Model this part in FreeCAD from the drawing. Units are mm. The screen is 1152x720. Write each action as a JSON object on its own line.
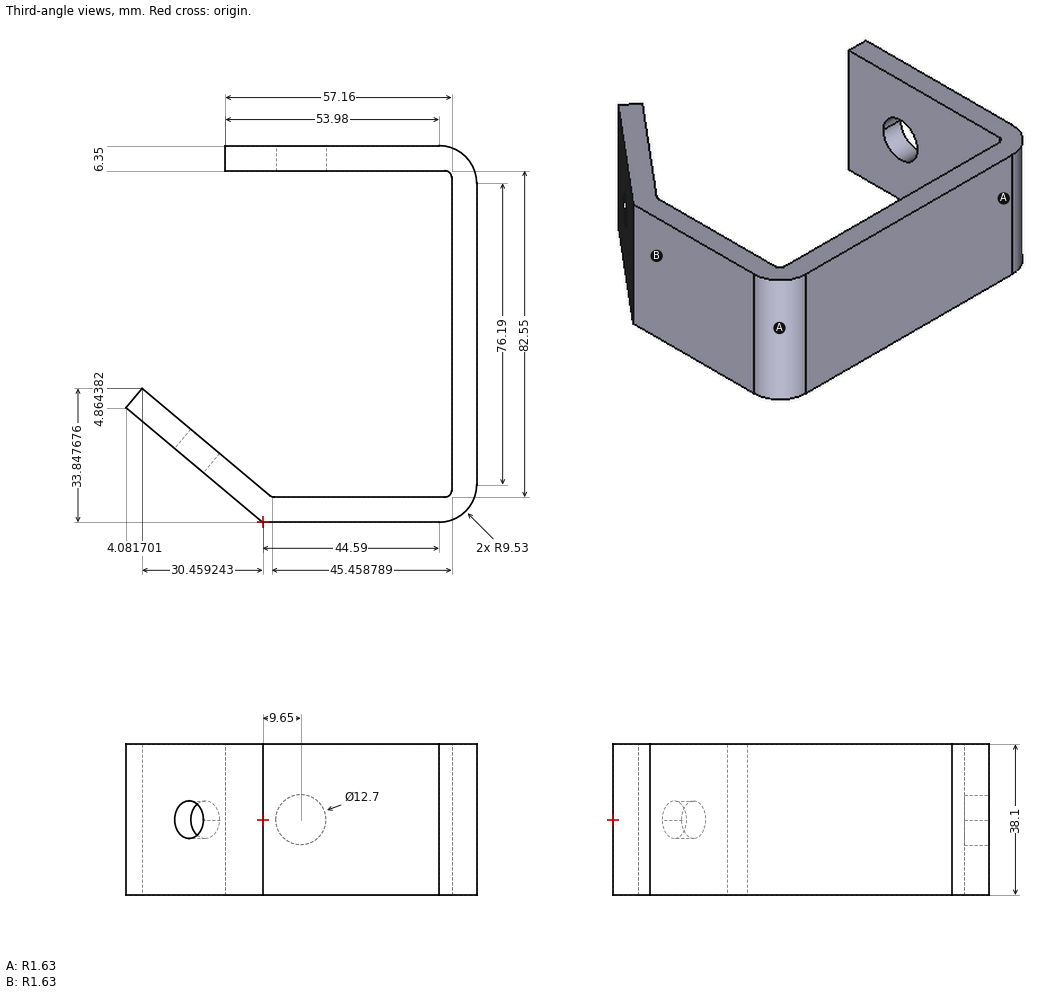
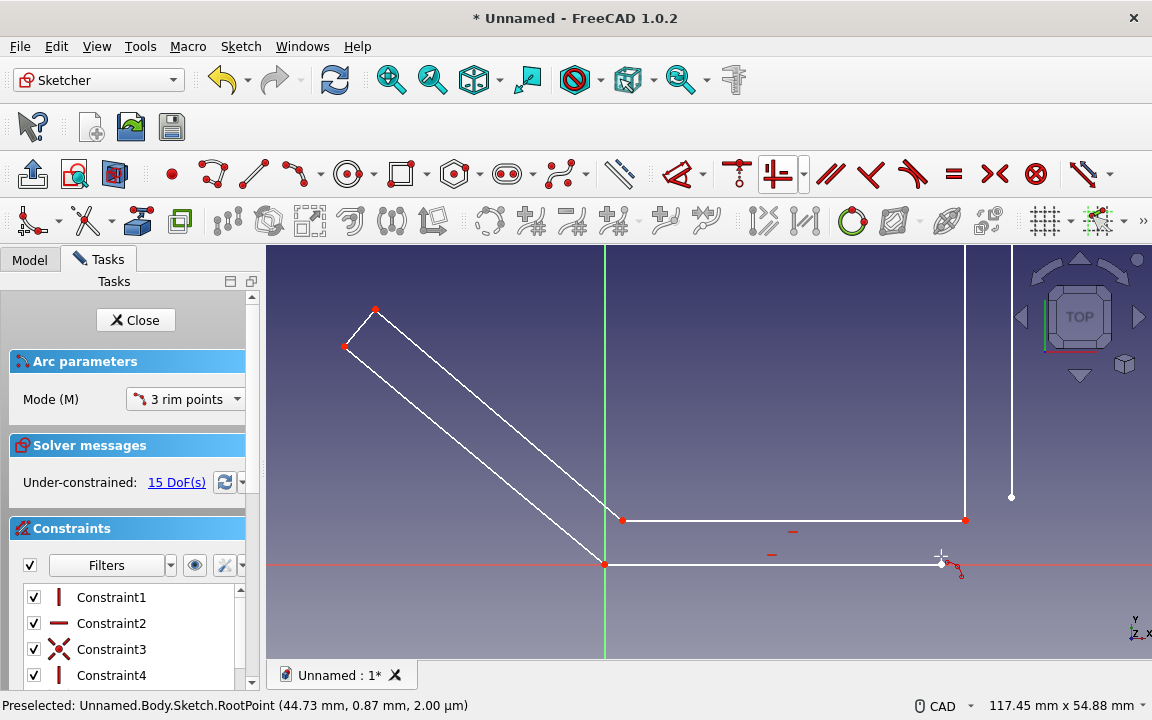
{"action": "scroll", "coordinate": [618, 596], "scroll_direction": "down", "scroll_amount": 5}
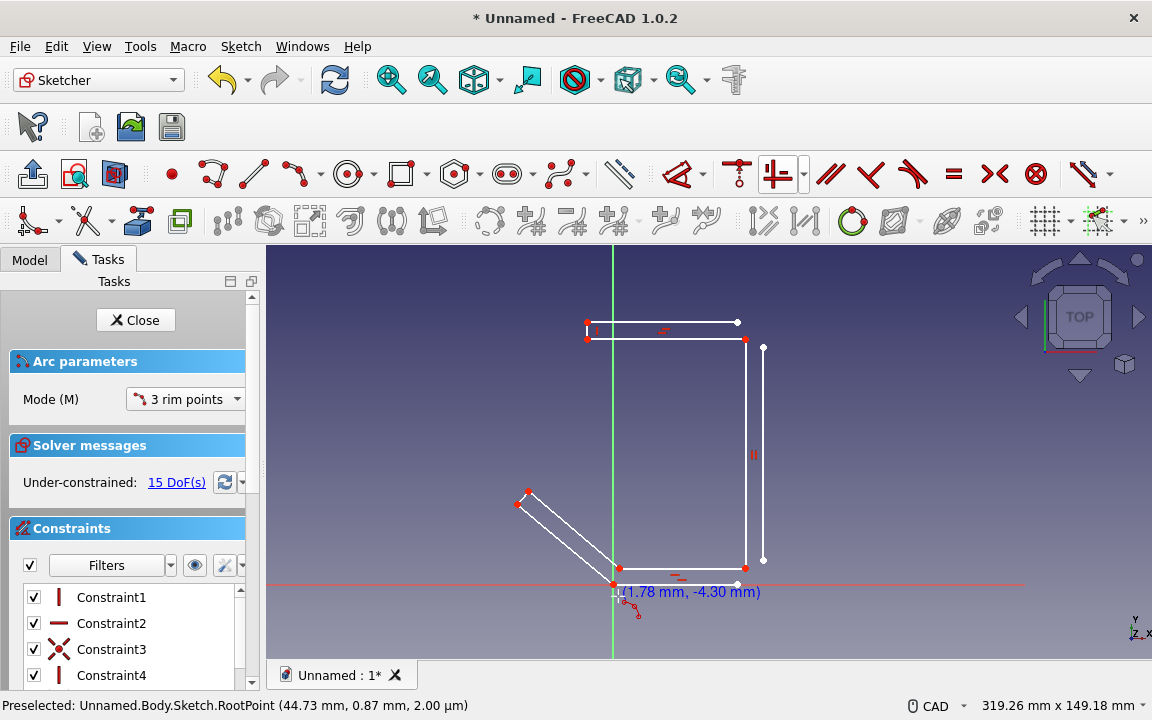
{"action": "left_click", "coordinate": [763, 348]}
{"action": "left_click", "coordinate": [737, 322]}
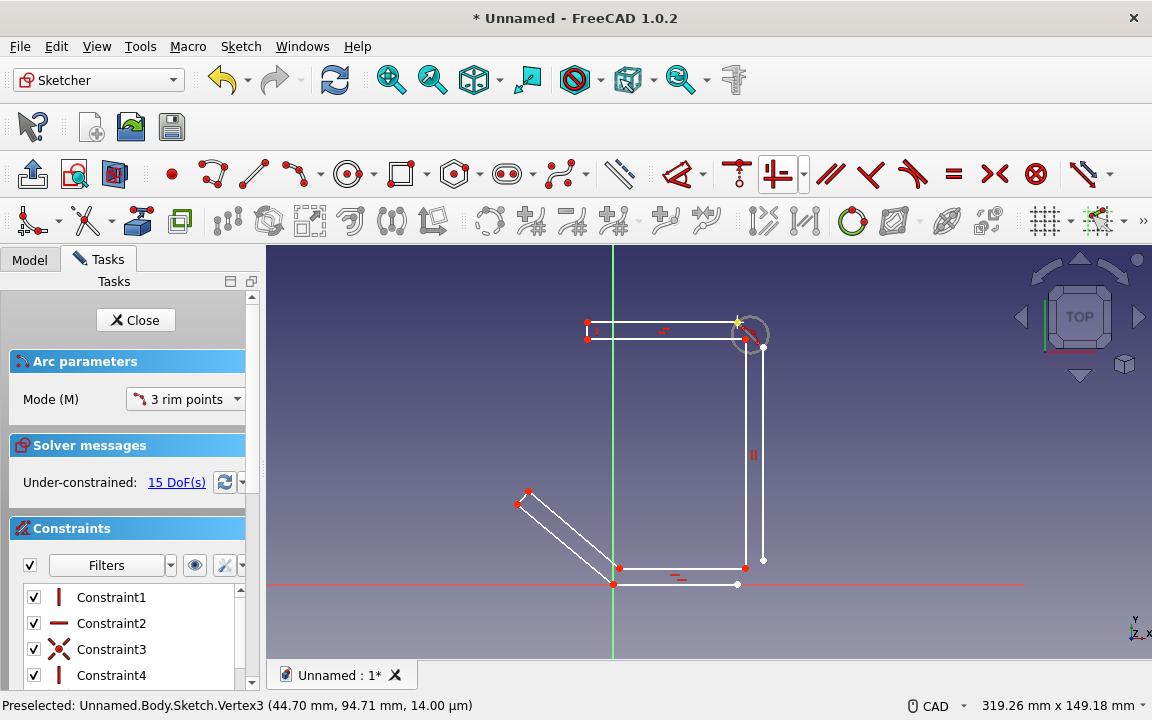
{"action": "scroll", "coordinate": [756, 328], "scroll_direction": "up", "scroll_amount": 4}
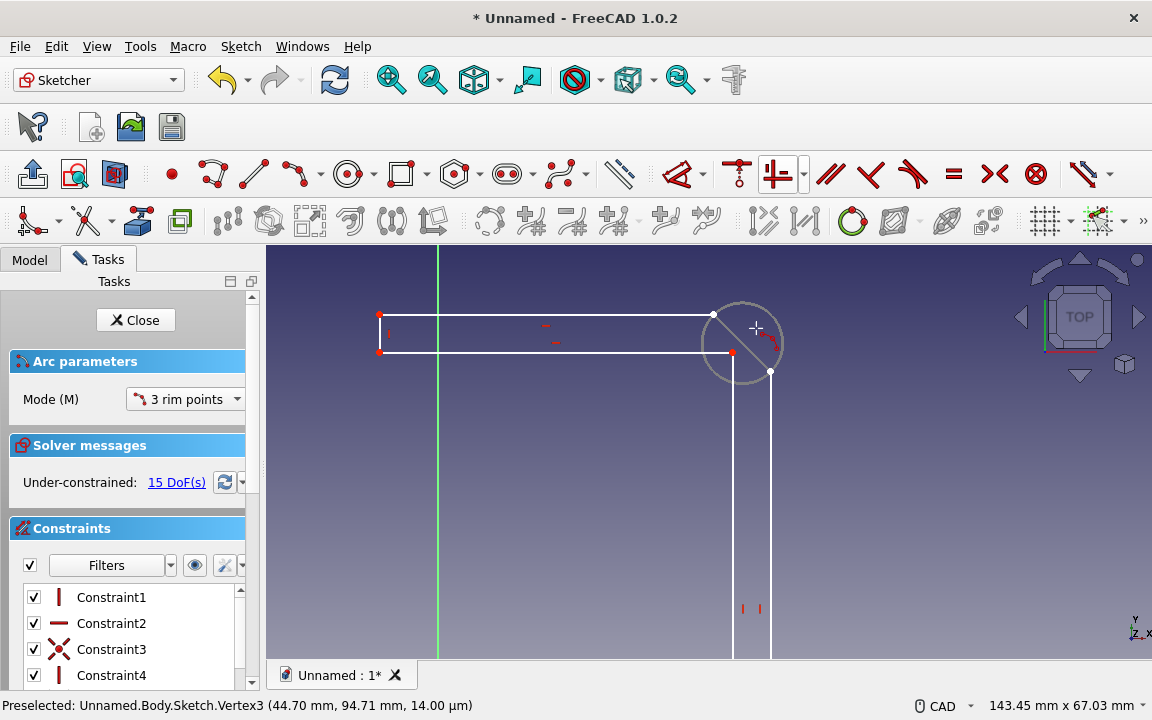
{"action": "left_click", "coordinate": [755, 329]}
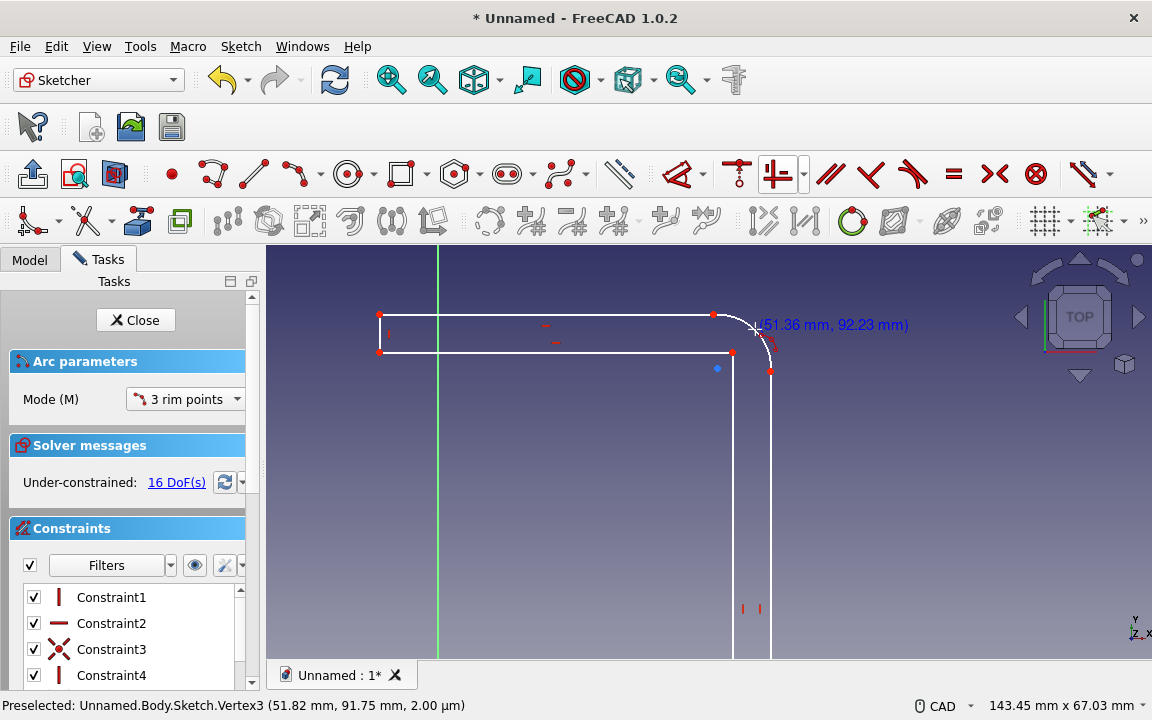
{"action": "scroll", "coordinate": [757, 327], "scroll_direction": "down", "scroll_amount": 4}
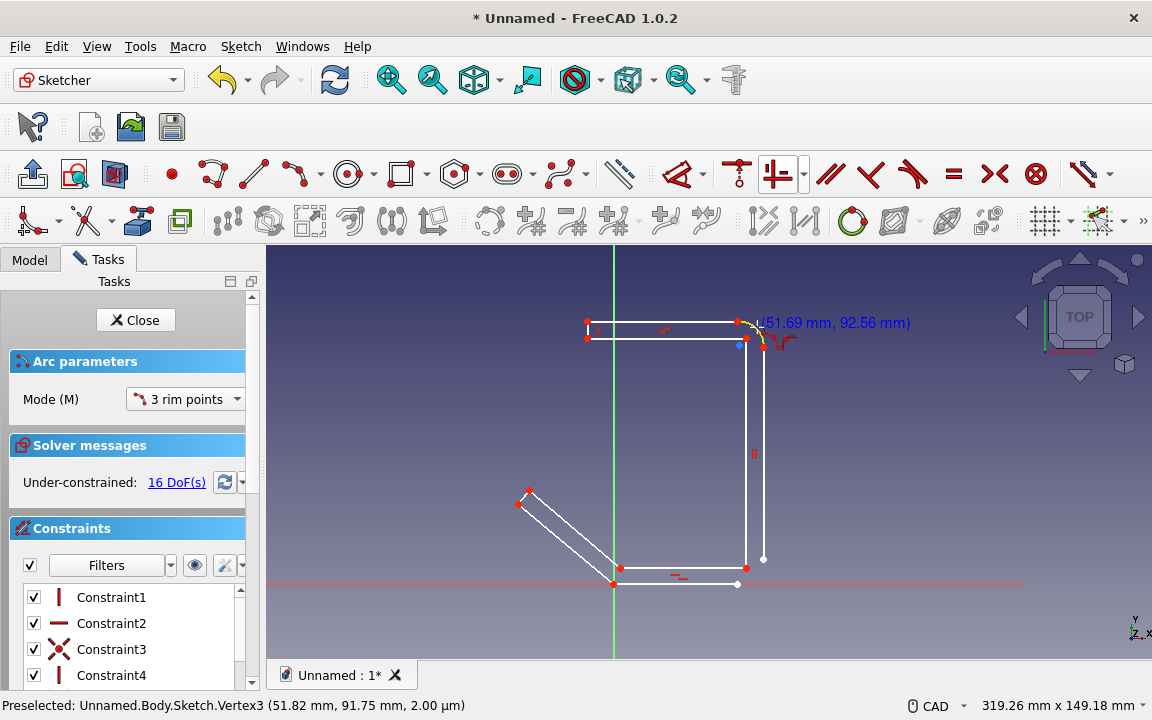
{"action": "left_click", "coordinate": [738, 584]}
{"action": "left_click", "coordinate": [764, 560]}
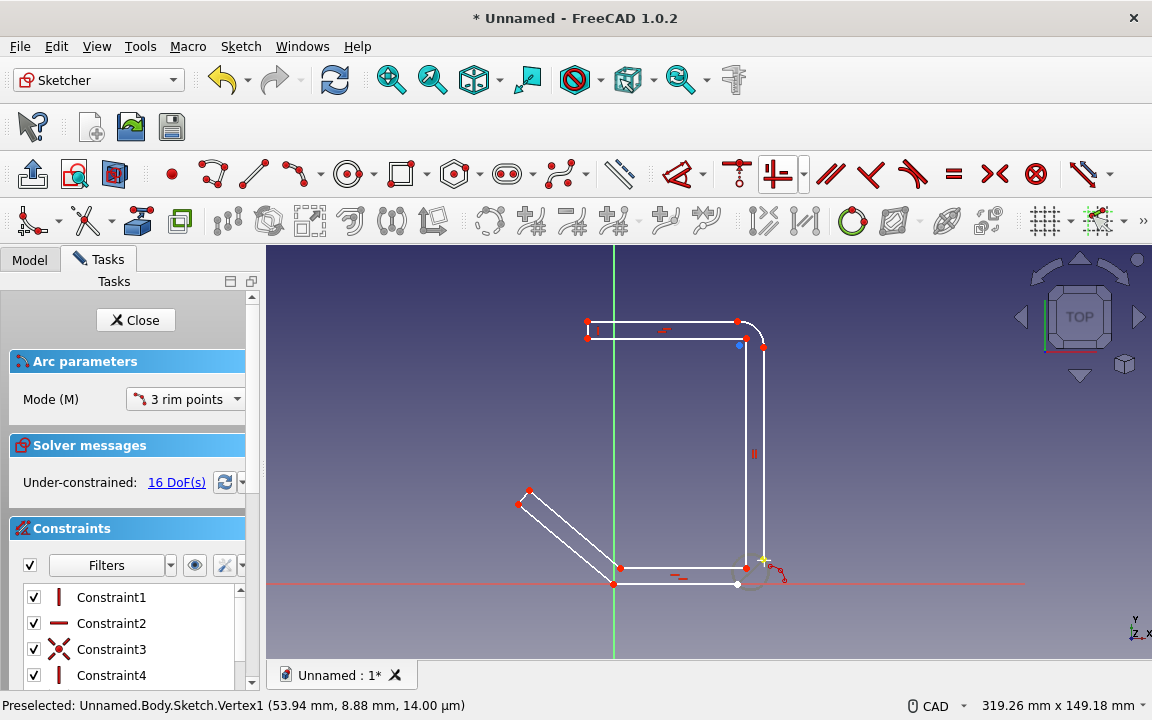
{"action": "scroll", "coordinate": [756, 577], "scroll_direction": "up", "scroll_amount": 4}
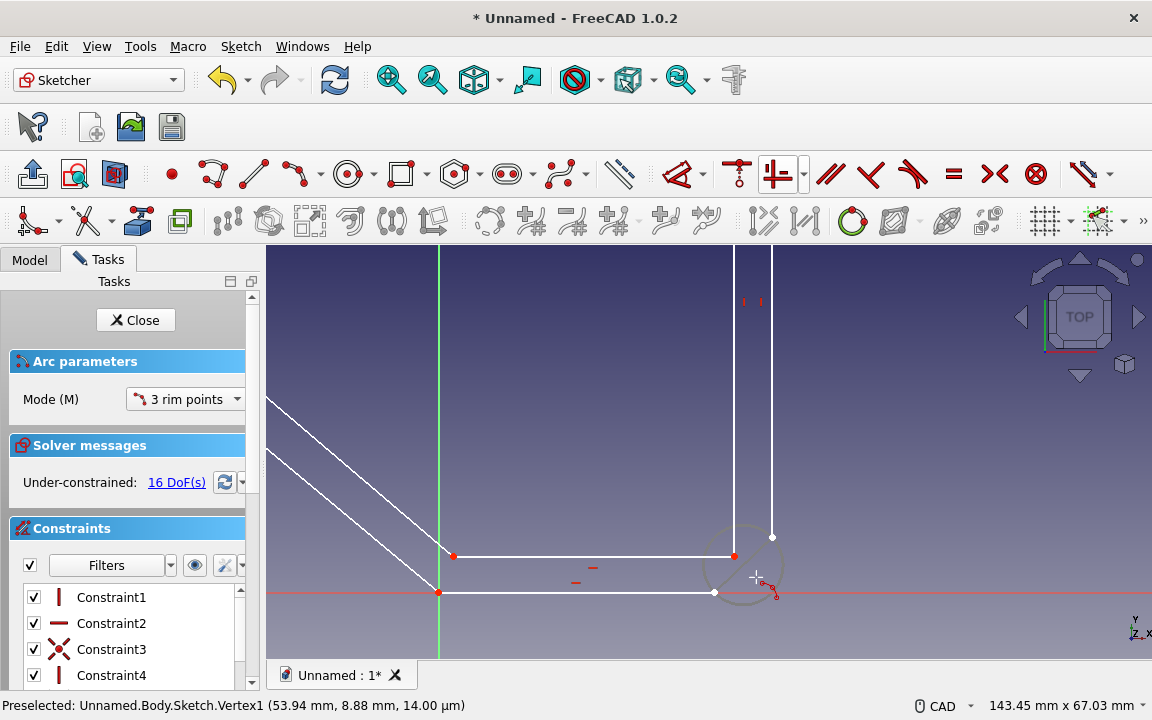
{"action": "left_click", "coordinate": [756, 575]}
{"action": "key", "text": "Escape"}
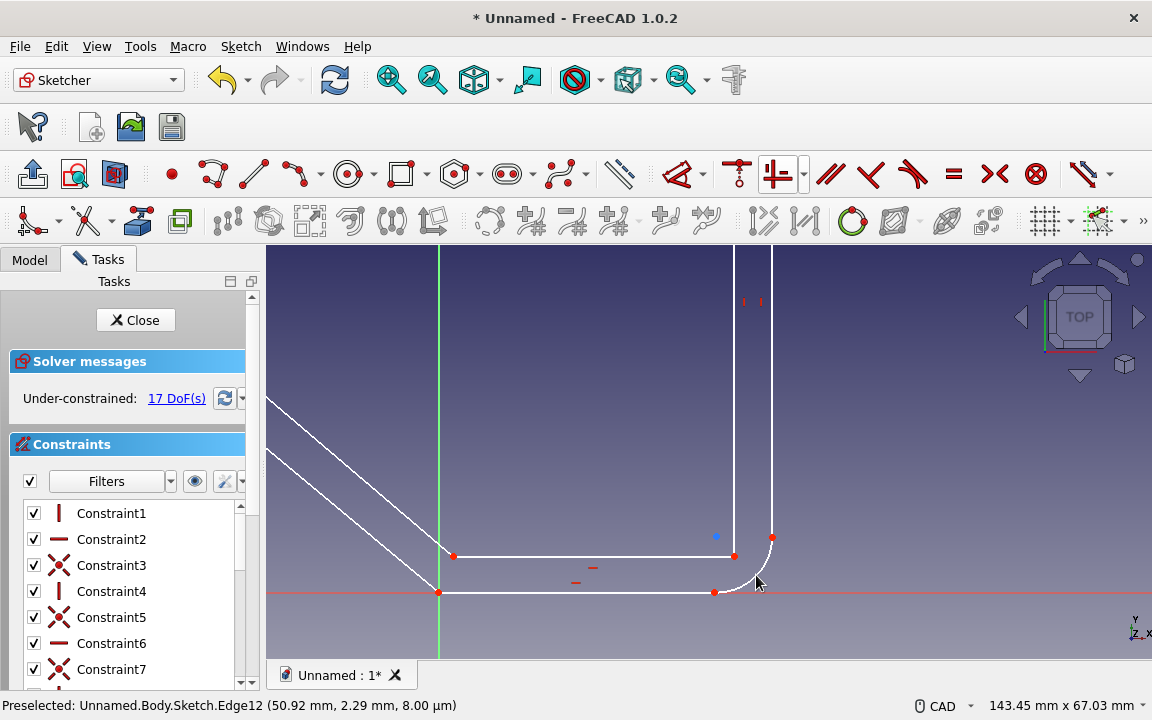
{"action": "left_click", "coordinate": [772, 396]}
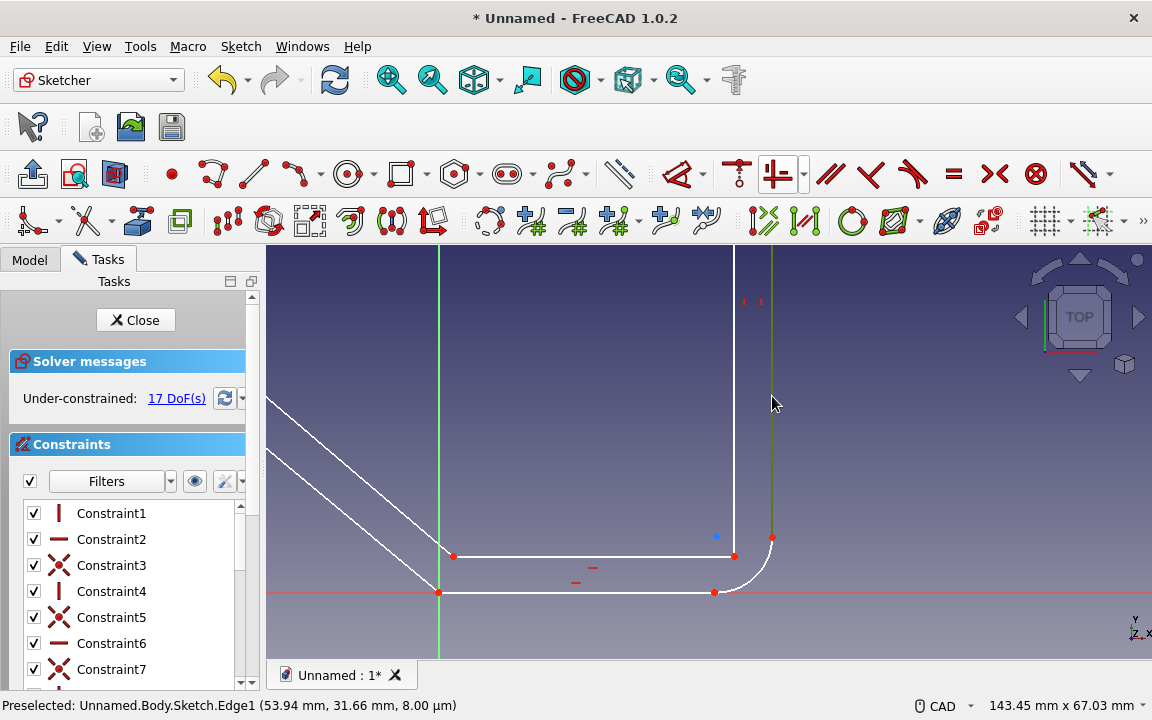
{"action": "scroll", "coordinate": [756, 577], "scroll_direction": "down", "scroll_amount": 4}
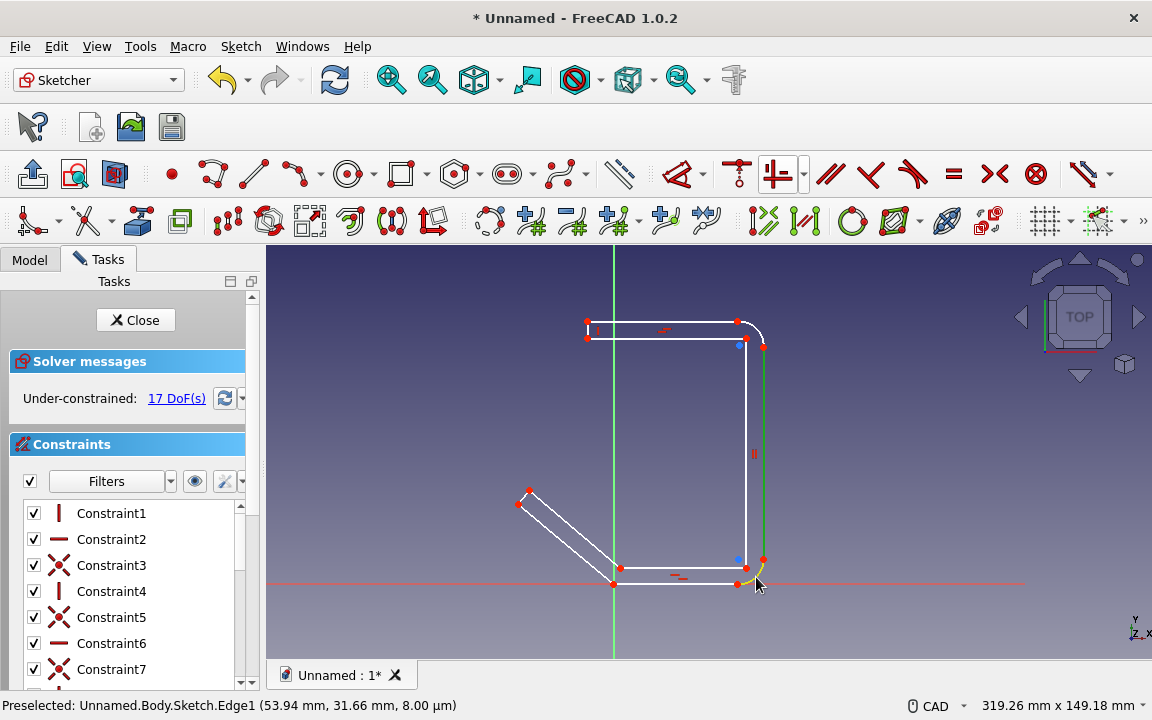
{"action": "left_click", "coordinate": [761, 335]}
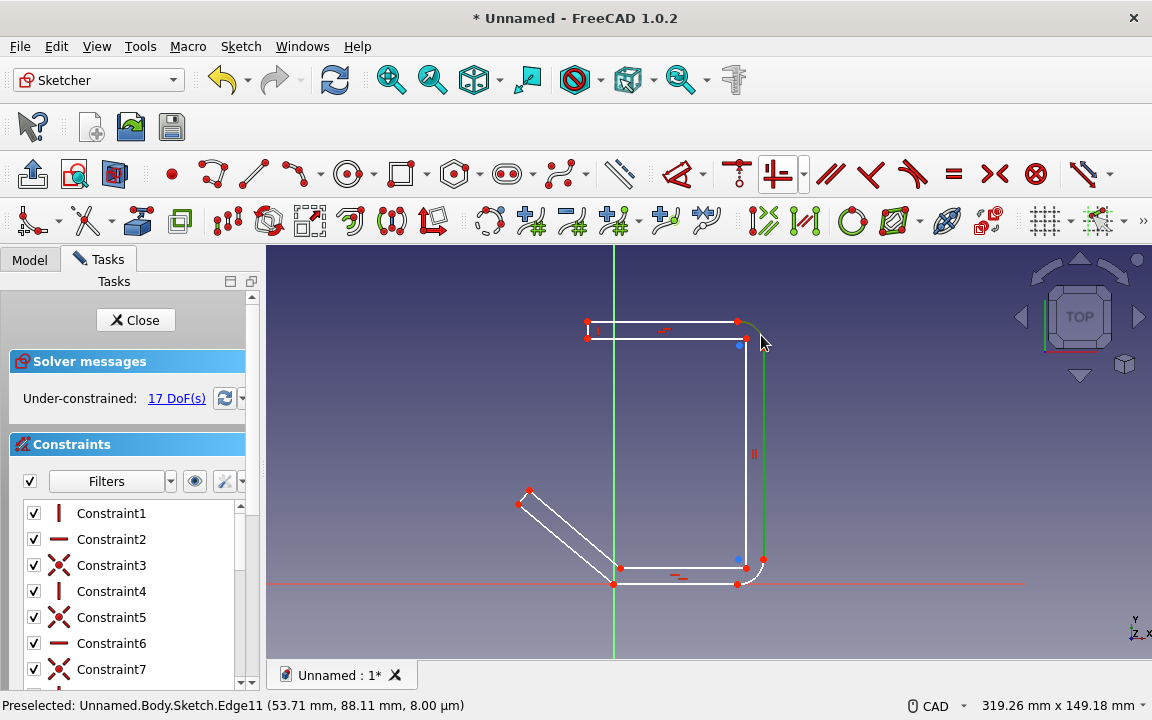
{"action": "key", "text": "t"}